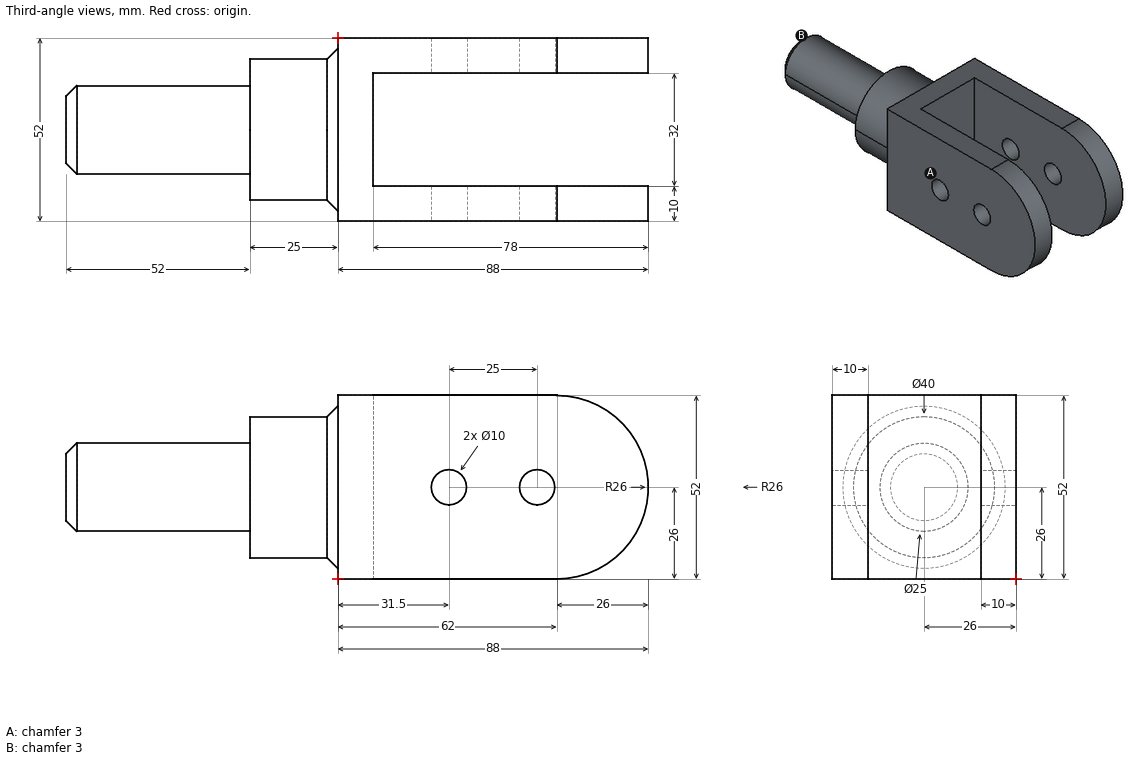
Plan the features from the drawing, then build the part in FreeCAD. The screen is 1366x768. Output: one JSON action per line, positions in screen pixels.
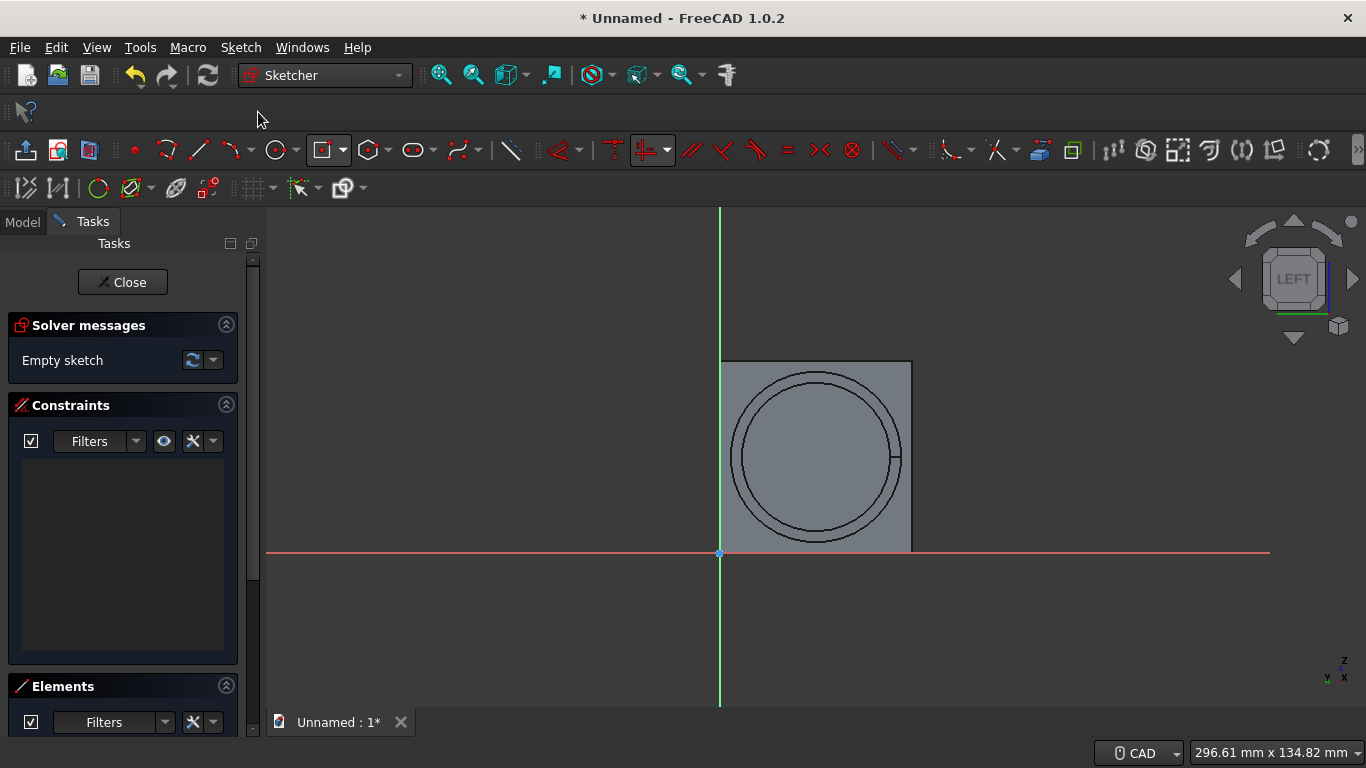
{"action": "scroll", "coordinate": [826, 502], "scroll_direction": "up", "scroll_amount": 4}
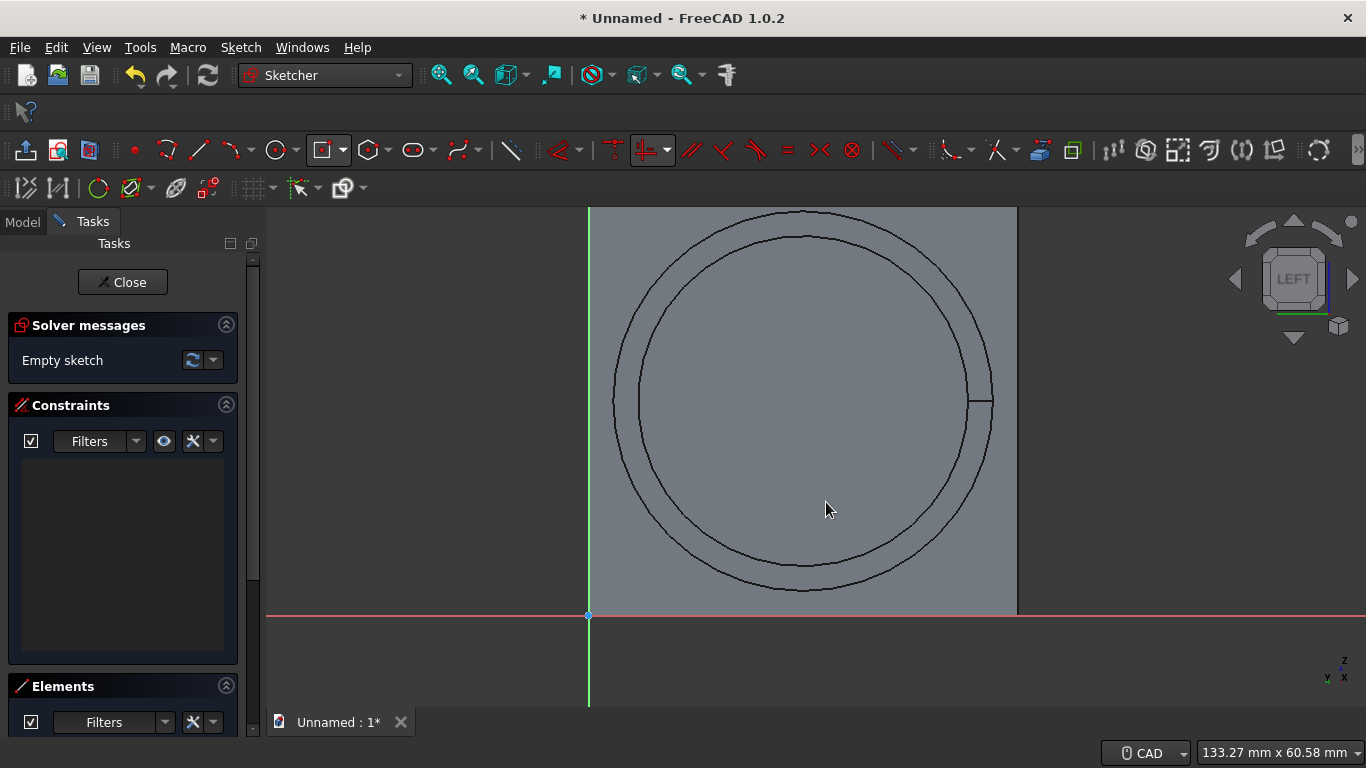
{"action": "left_click", "coordinate": [276, 150]}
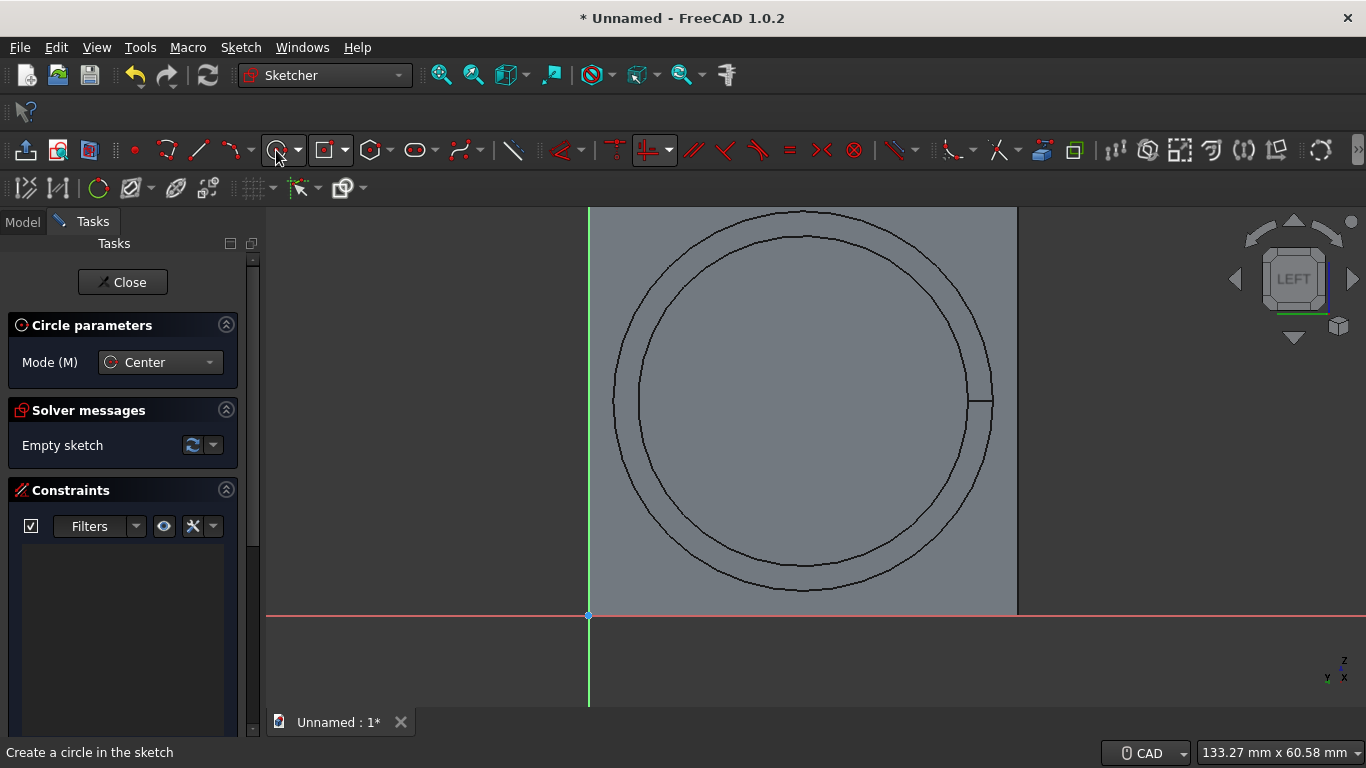
{"action": "left_click", "coordinate": [803, 401]}
{"action": "left_click", "coordinate": [876, 328]}
{"action": "key", "text": "Escape"}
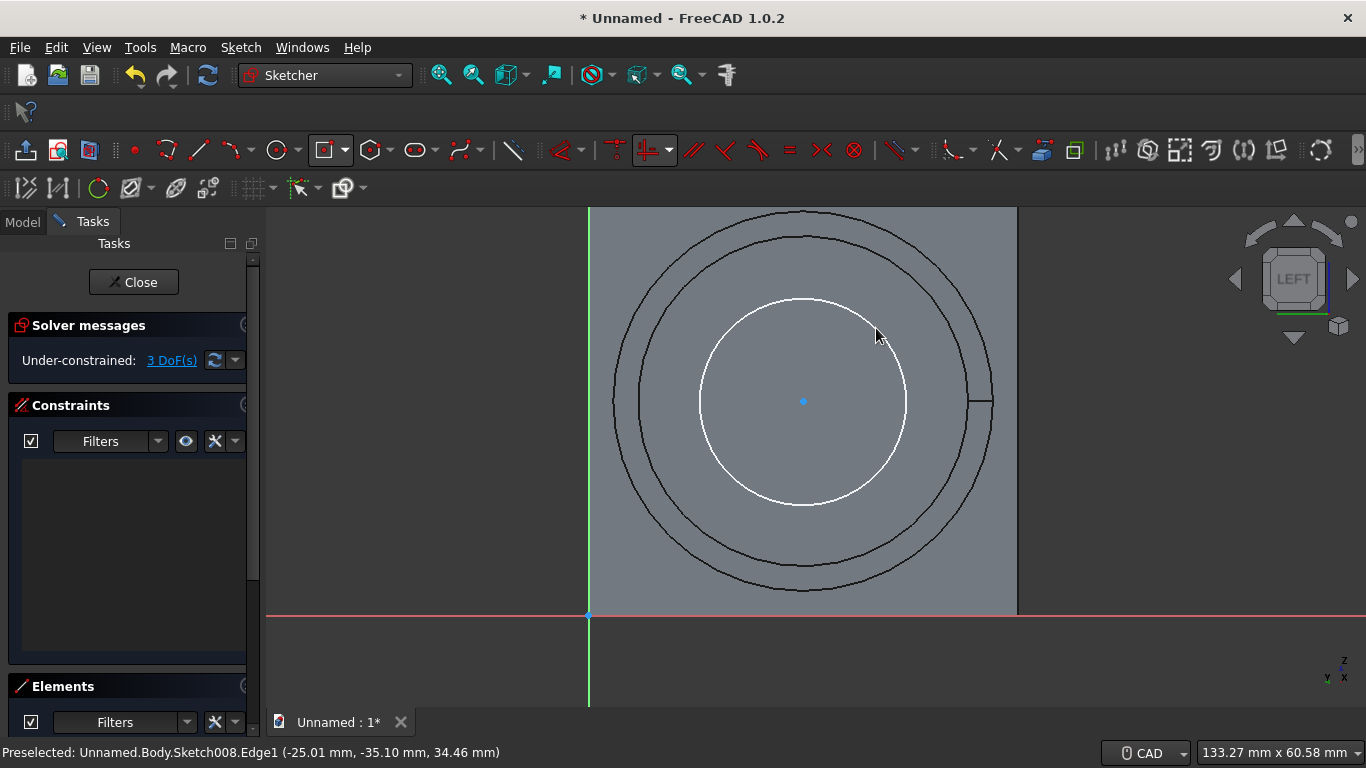
{"action": "left_click", "coordinate": [560, 150]}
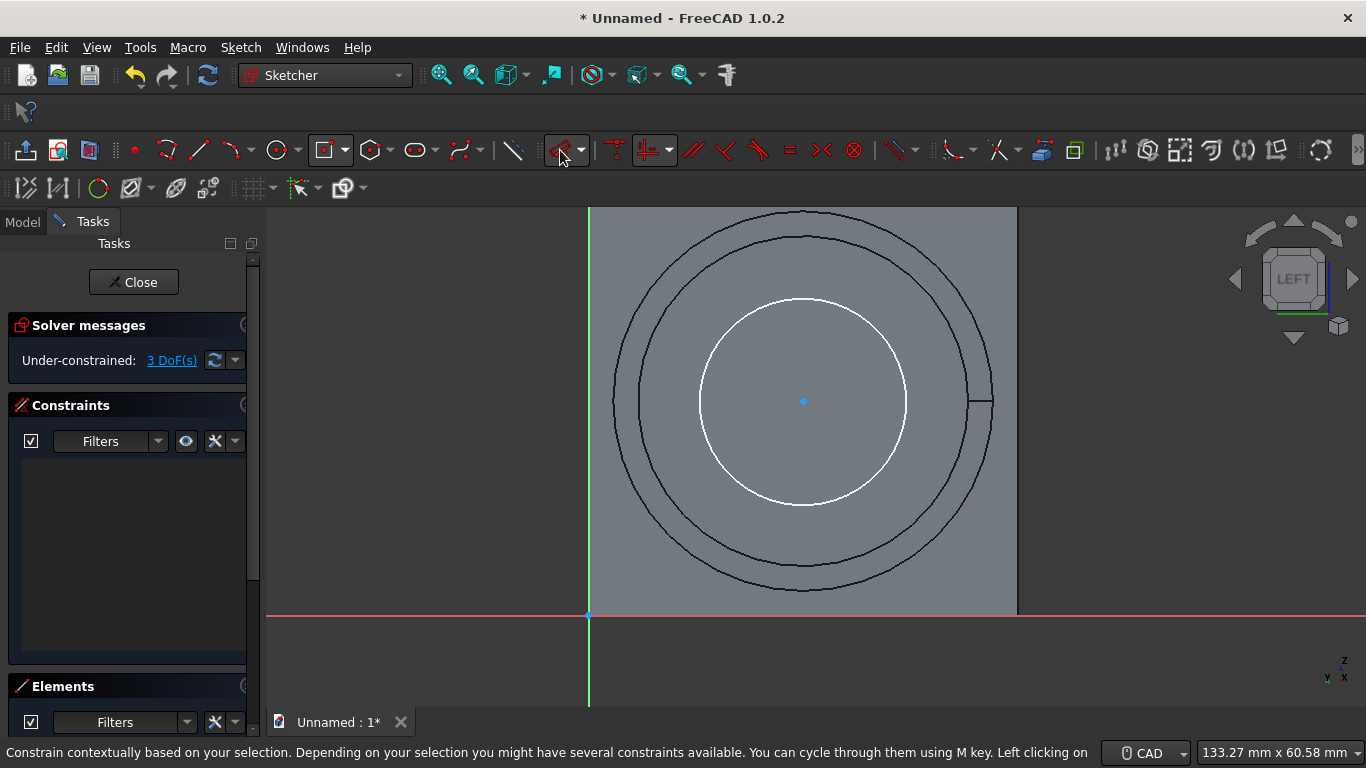
{"action": "left_click", "coordinate": [876, 329]}
{"action": "left_click", "coordinate": [899, 306]}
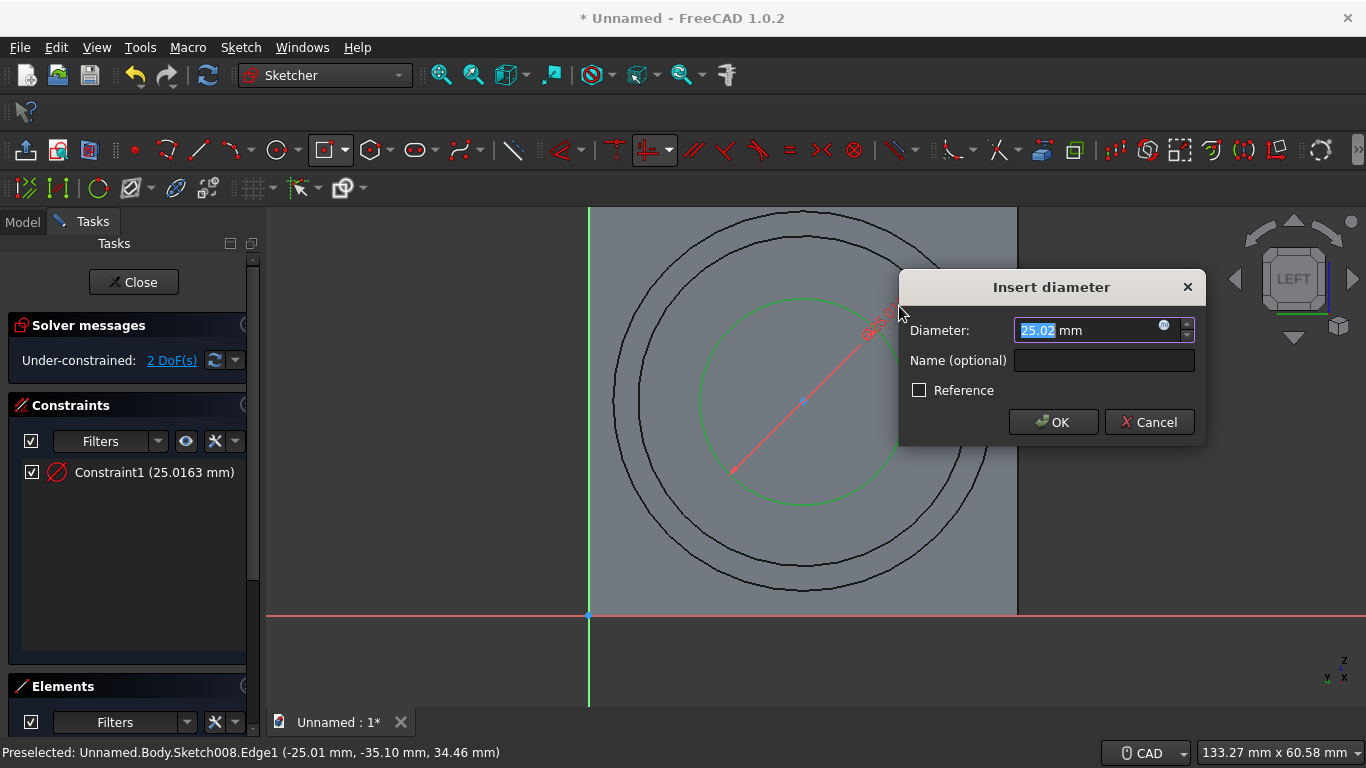
{"action": "type", "text": "25"}
{"action": "key", "text": "Return"}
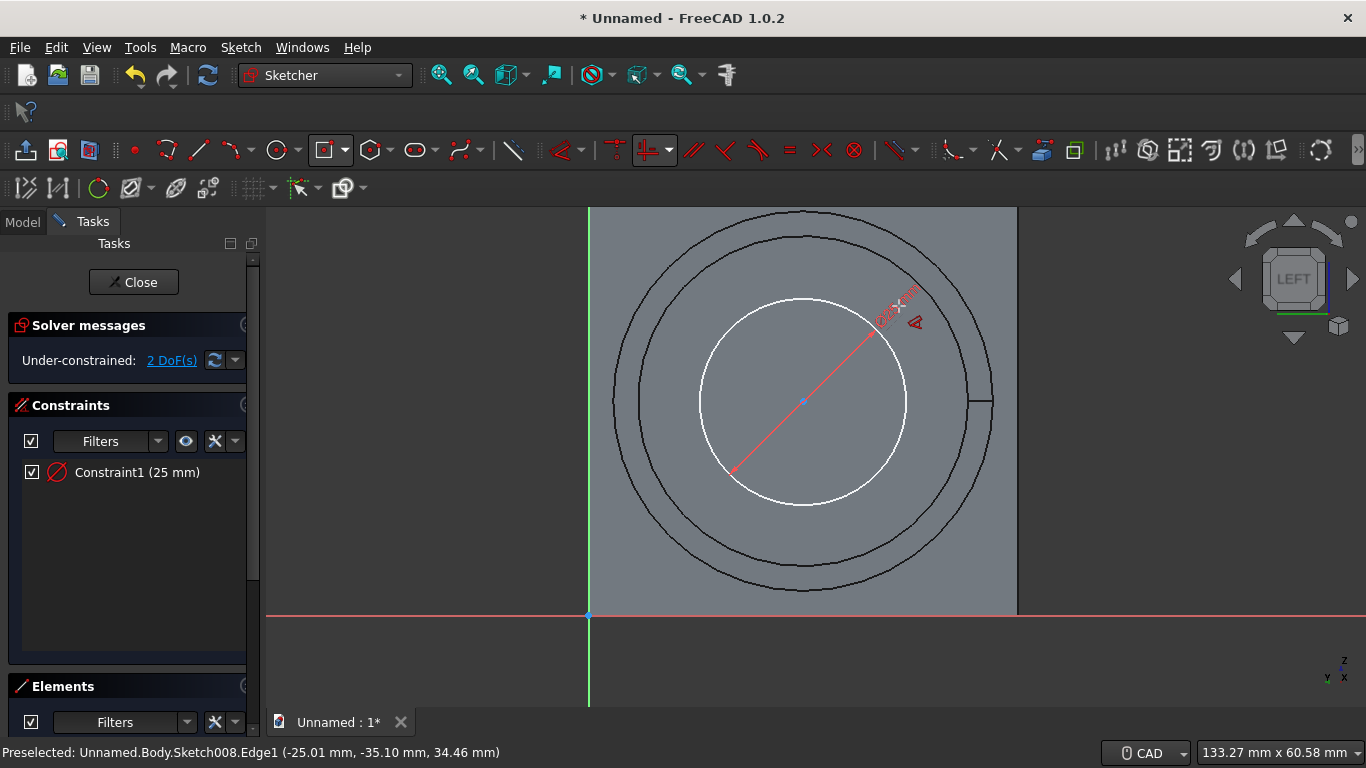
{"action": "left_click", "coordinate": [803, 402]}
{"action": "left_click", "coordinate": [696, 650]}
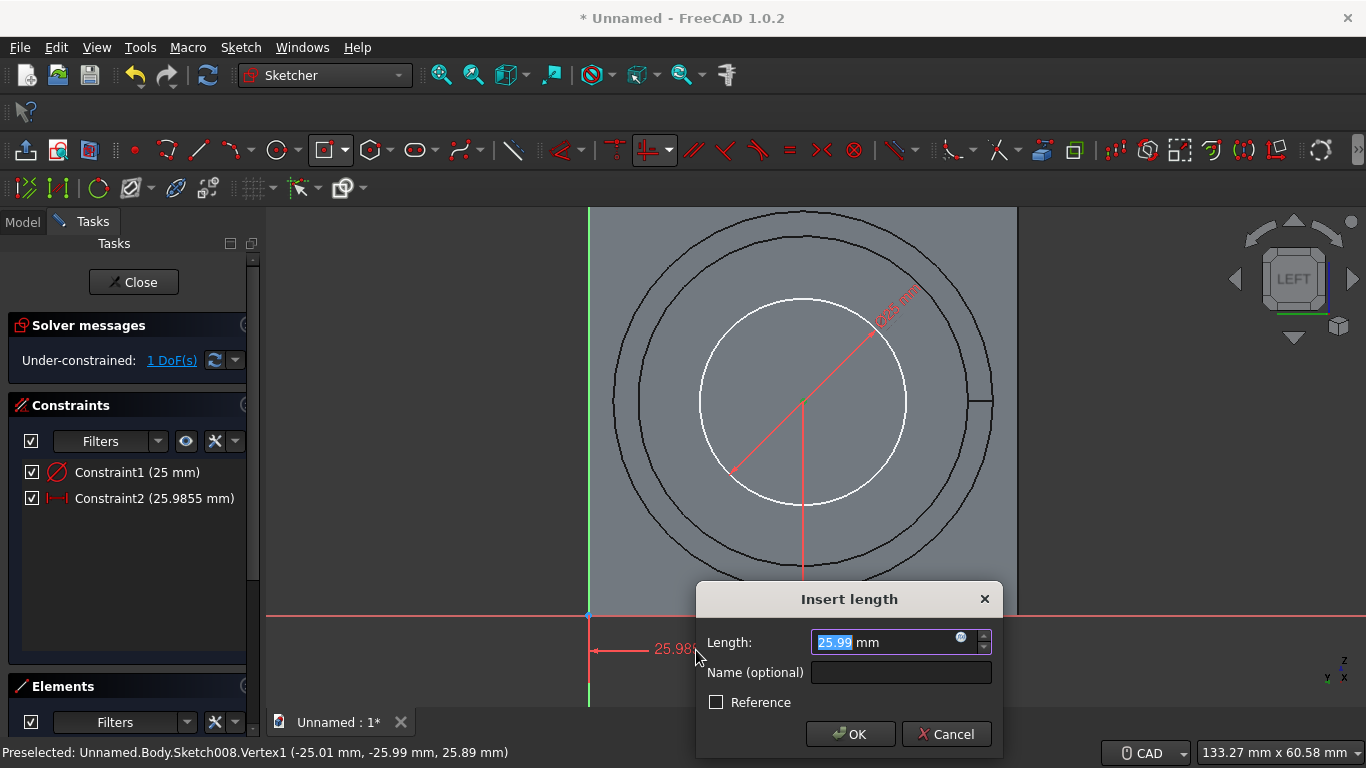
{"action": "type", "text": "26"}
{"action": "key", "text": "Return"}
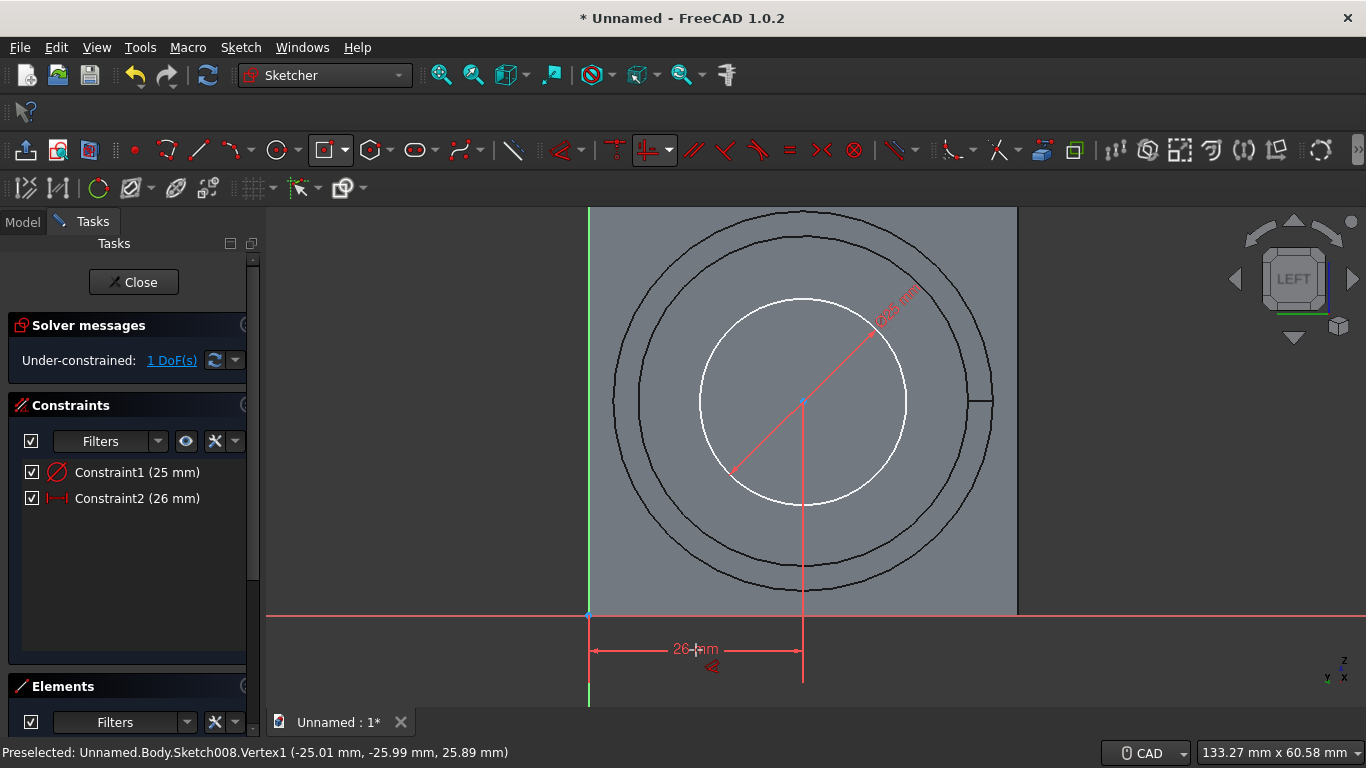
{"action": "left_click", "coordinate": [803, 402]}
{"action": "left_click", "coordinate": [555, 509]}